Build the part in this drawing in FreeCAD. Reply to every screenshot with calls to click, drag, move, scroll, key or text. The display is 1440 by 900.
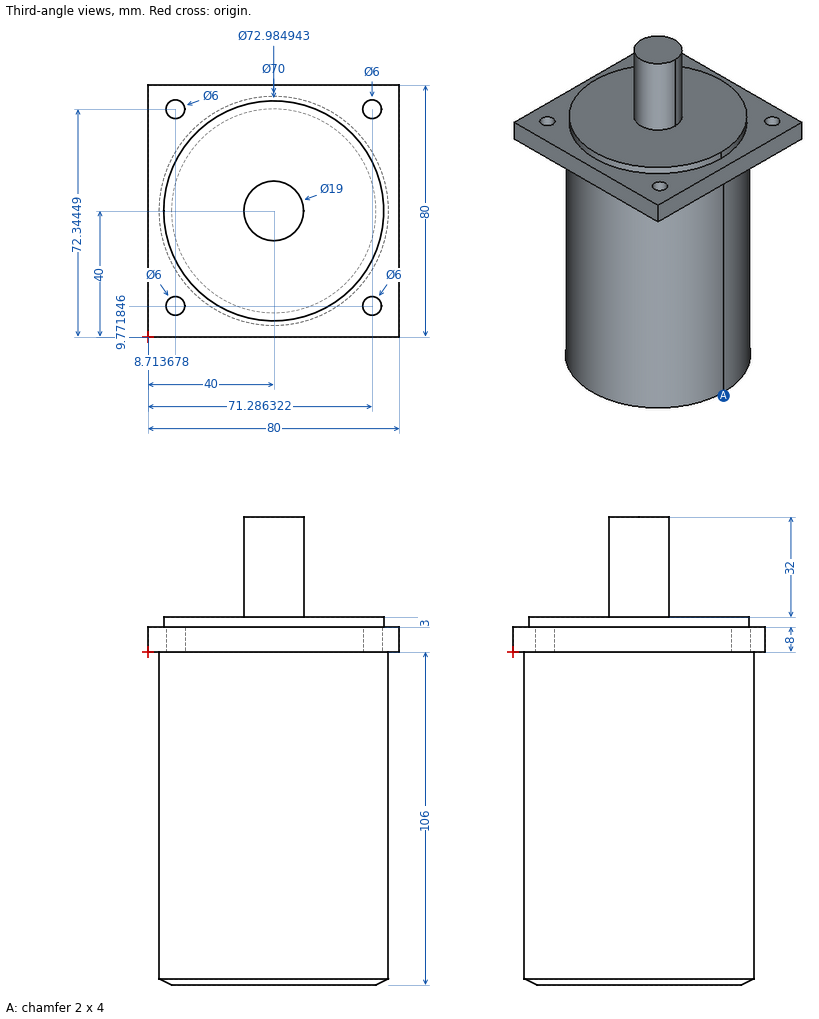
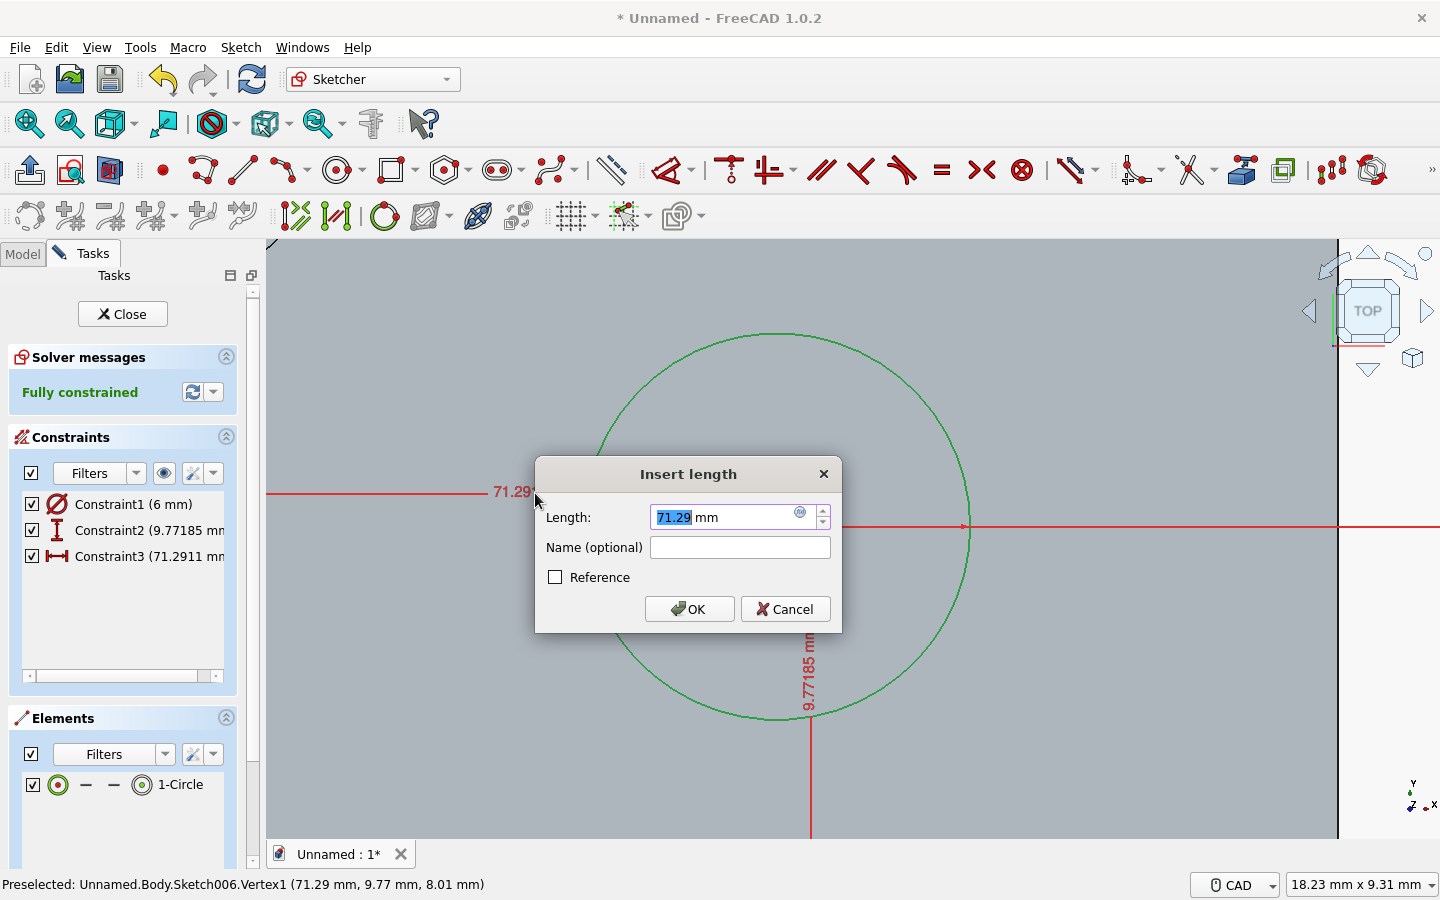
text(71.286322)
key(Return)
key(Escape)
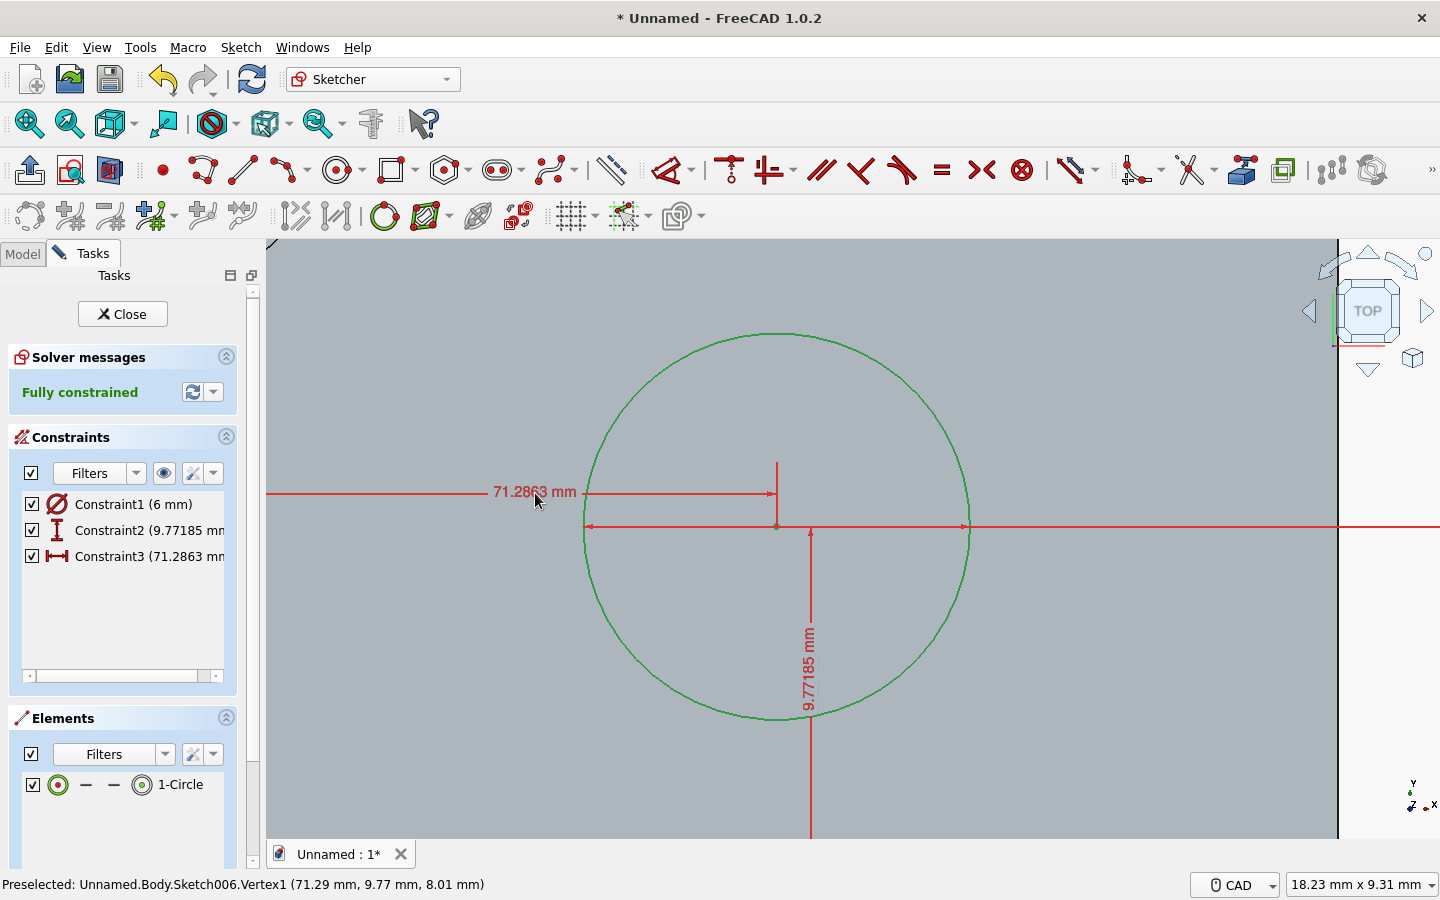
click(123, 314)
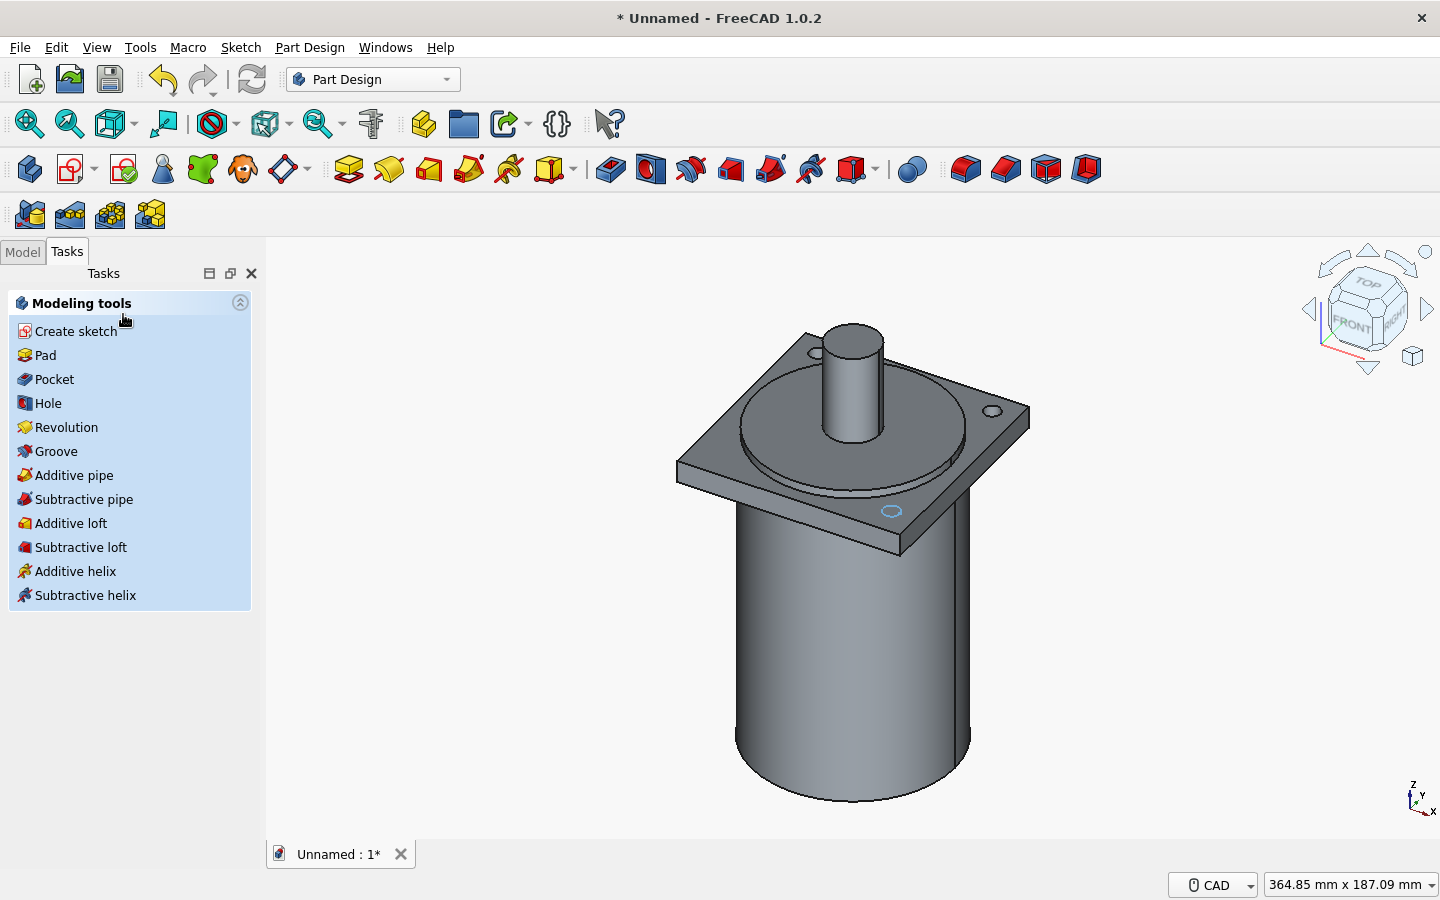
click(612, 170)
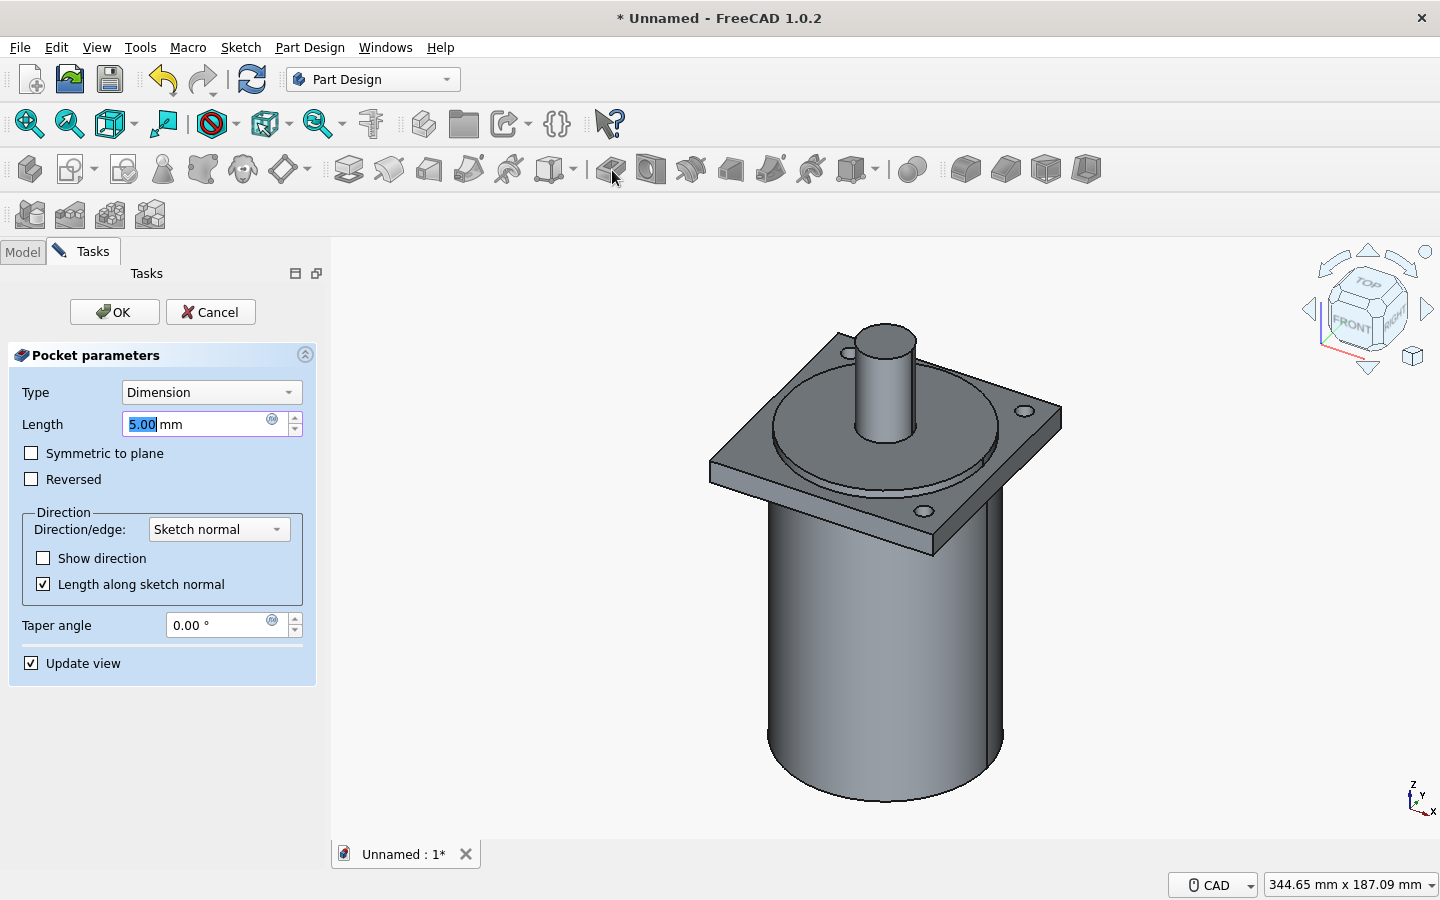
click(212, 392)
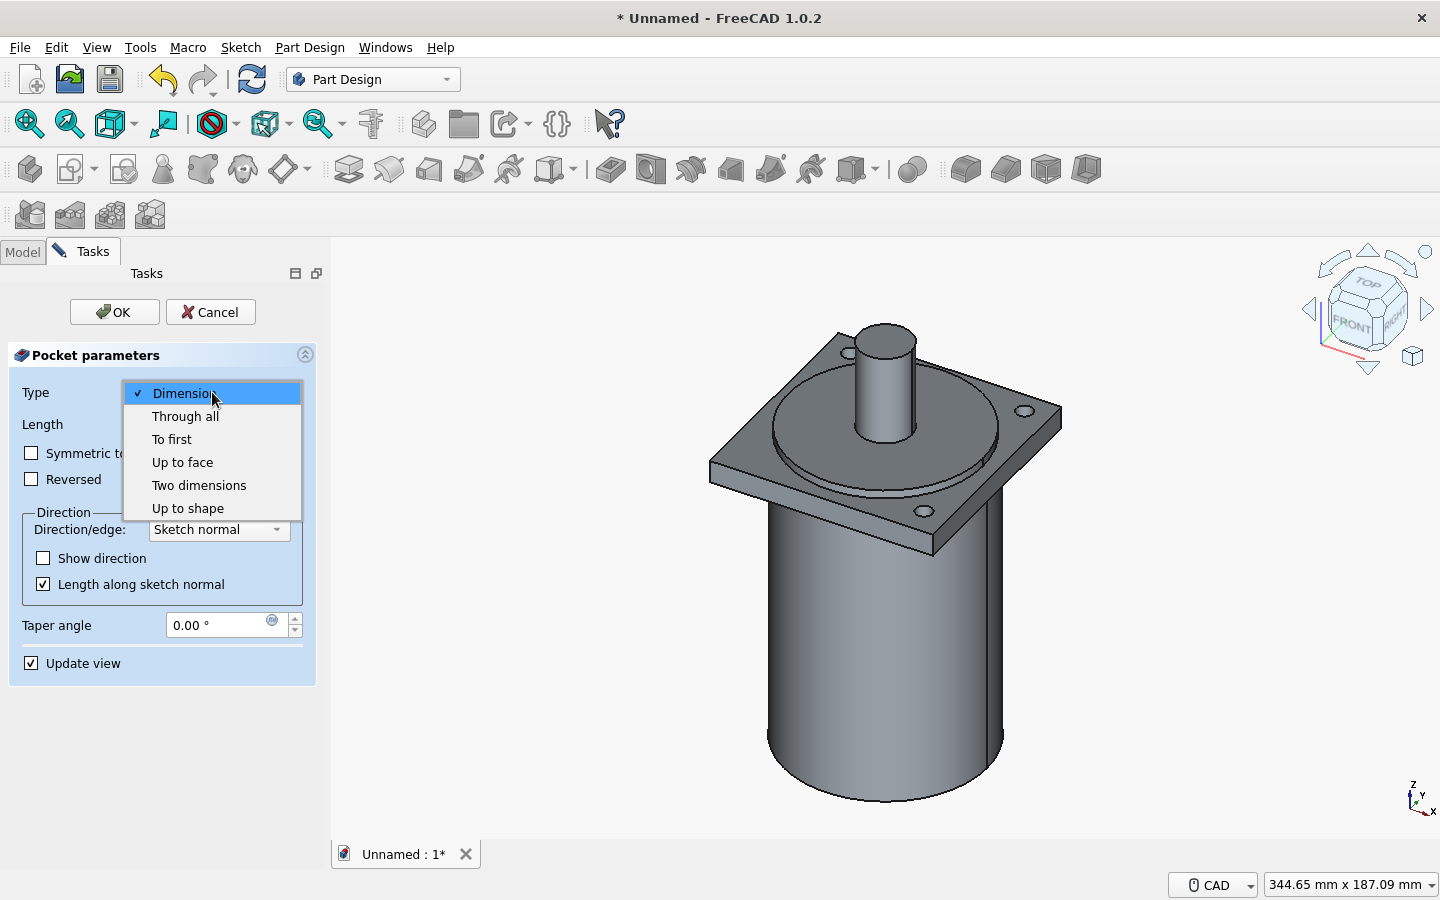
click(212, 440)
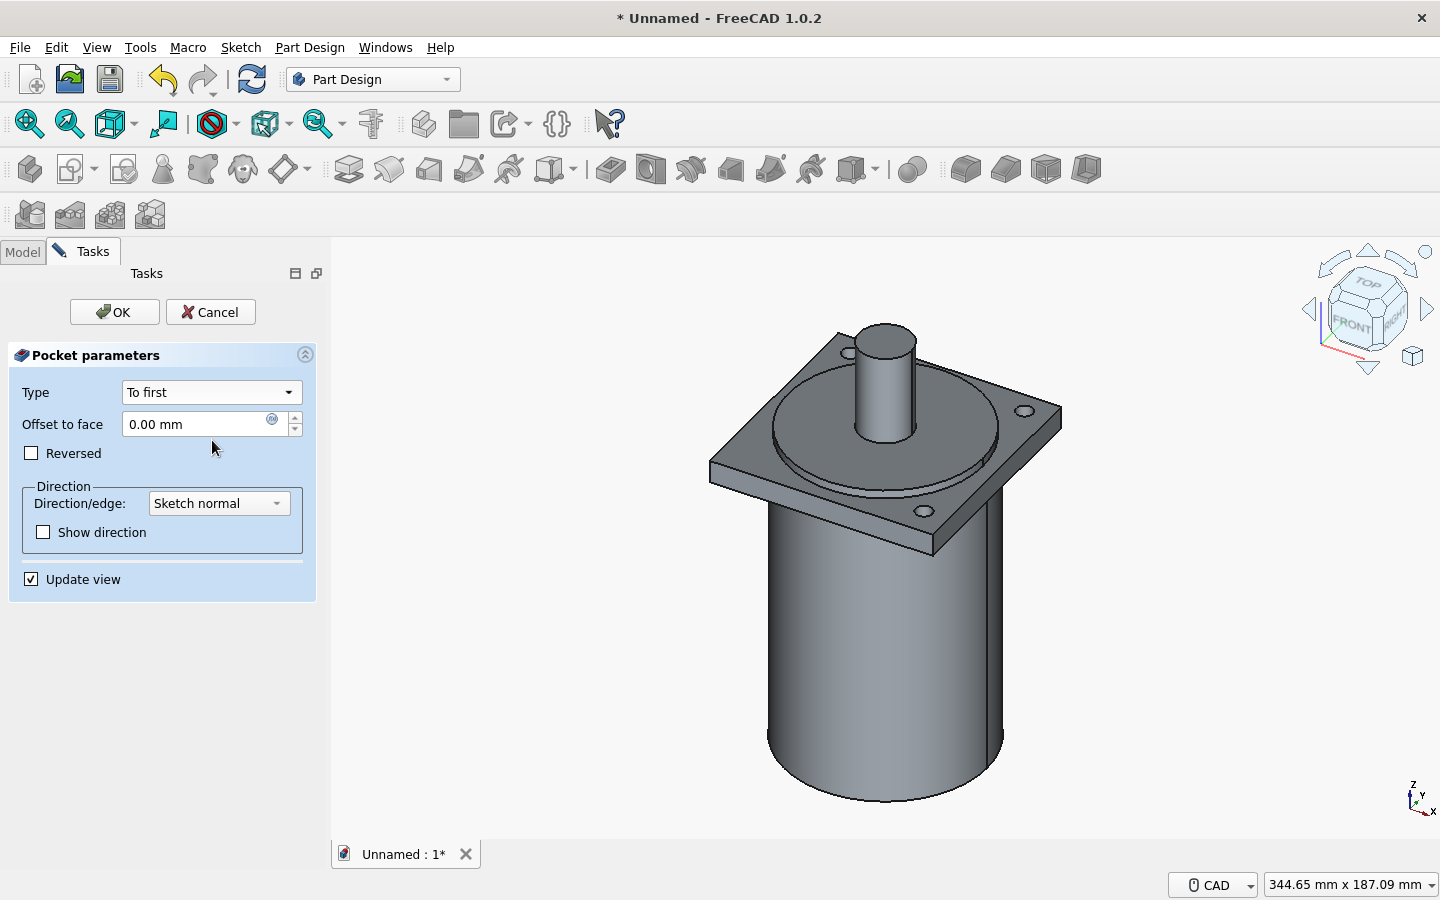
click(115, 312)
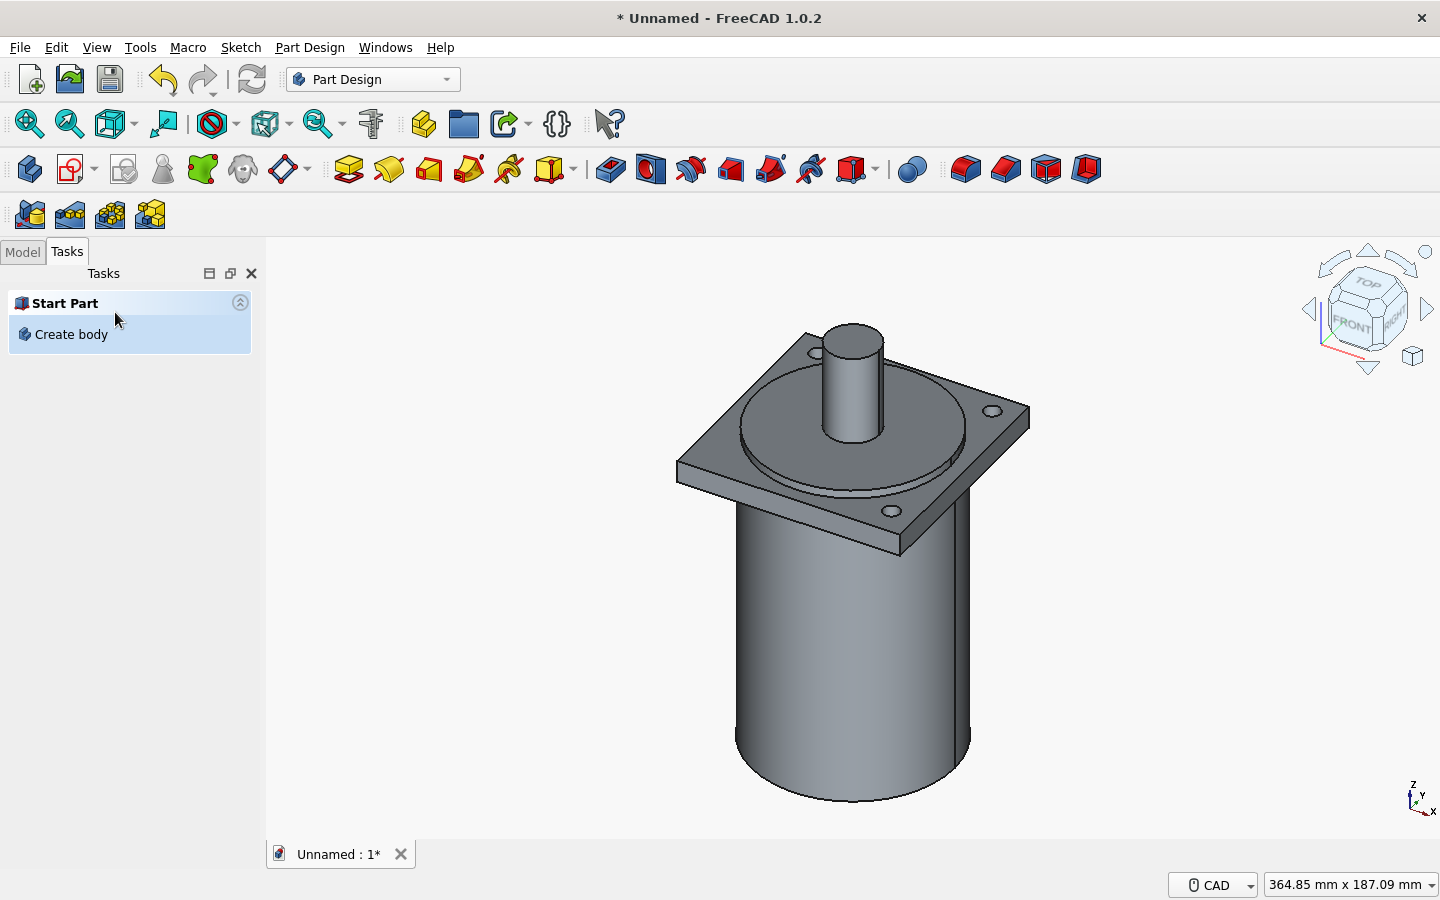
click(862, 509)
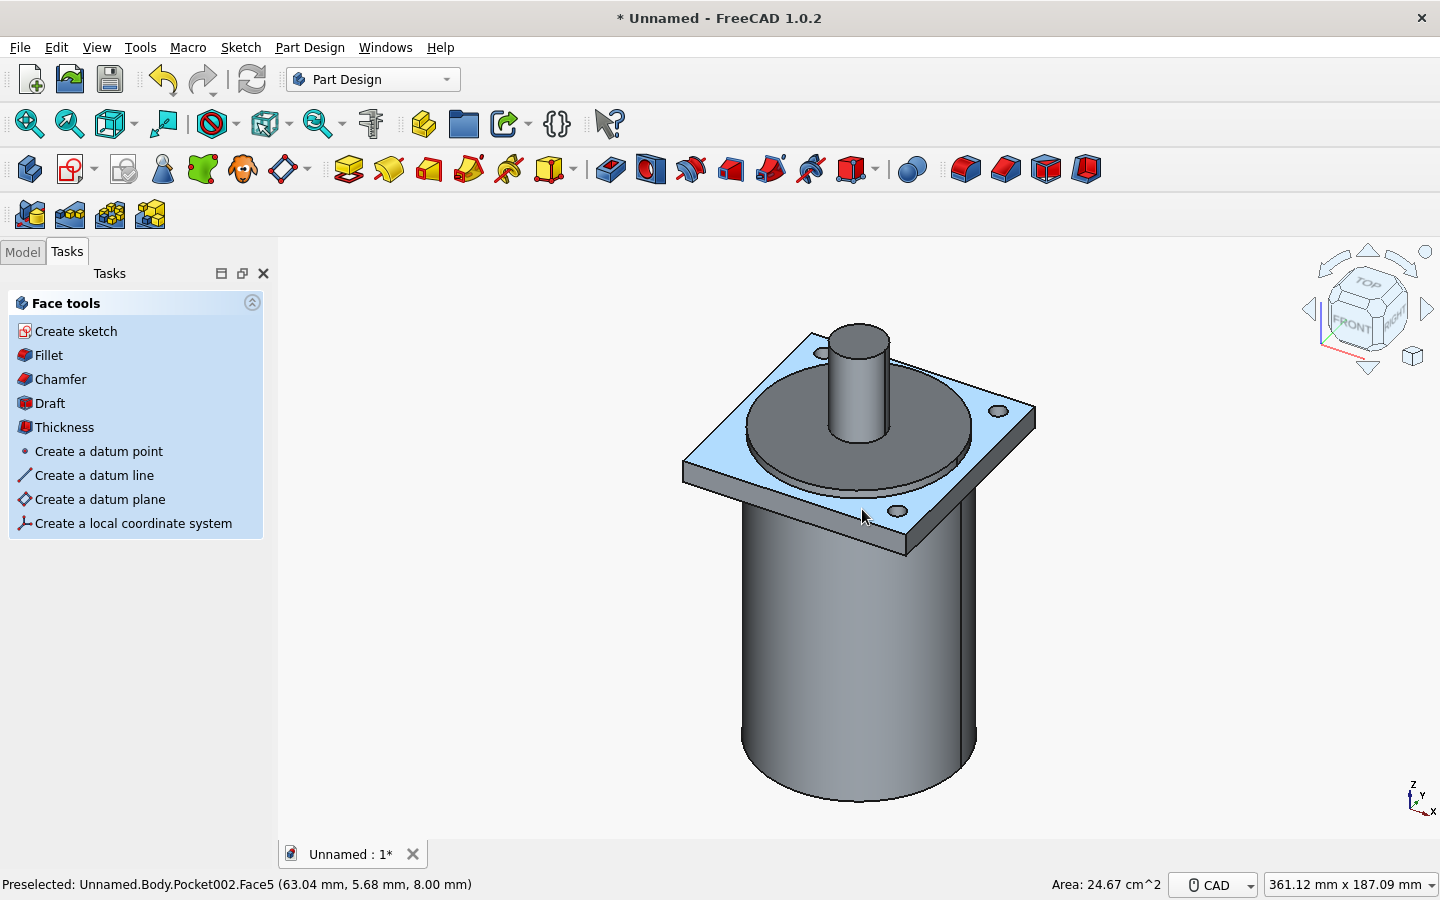
click(70, 170)